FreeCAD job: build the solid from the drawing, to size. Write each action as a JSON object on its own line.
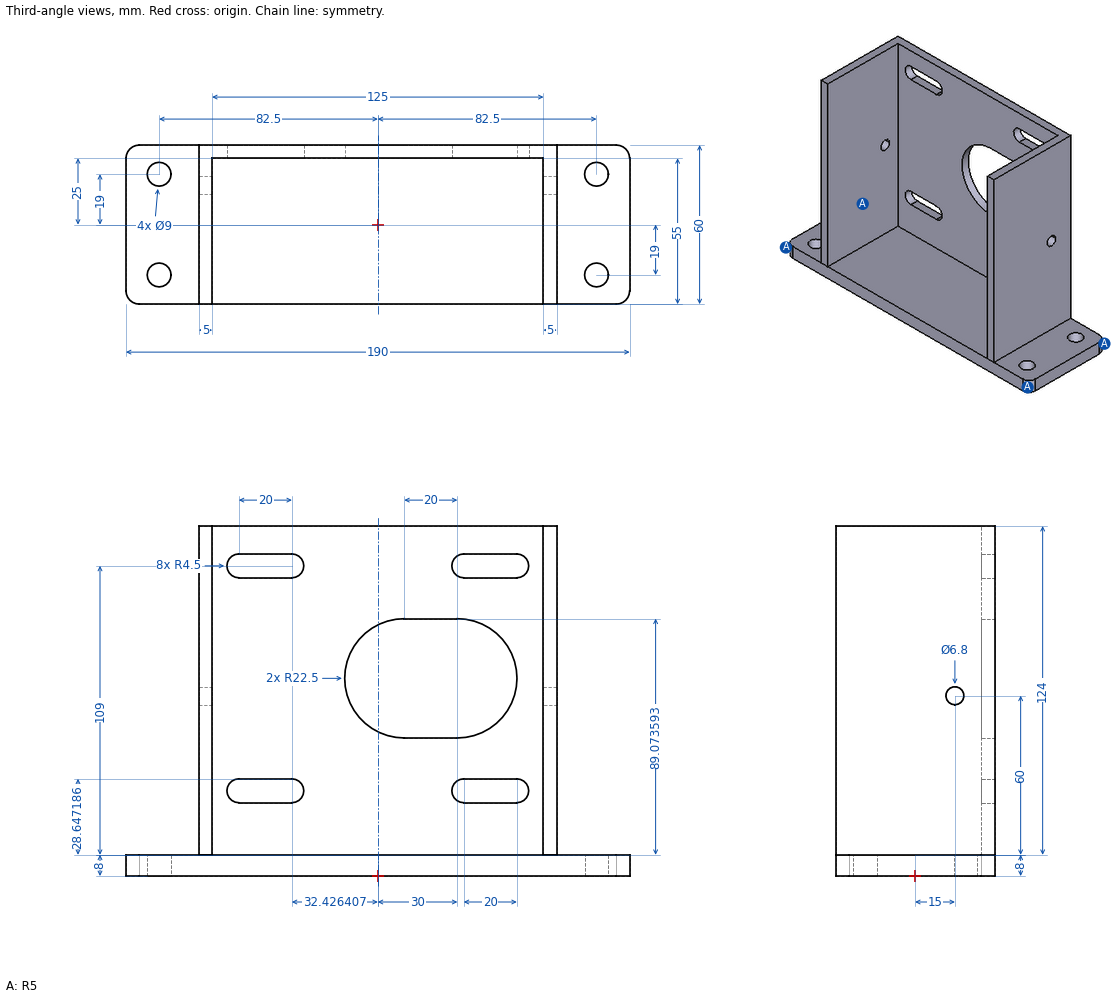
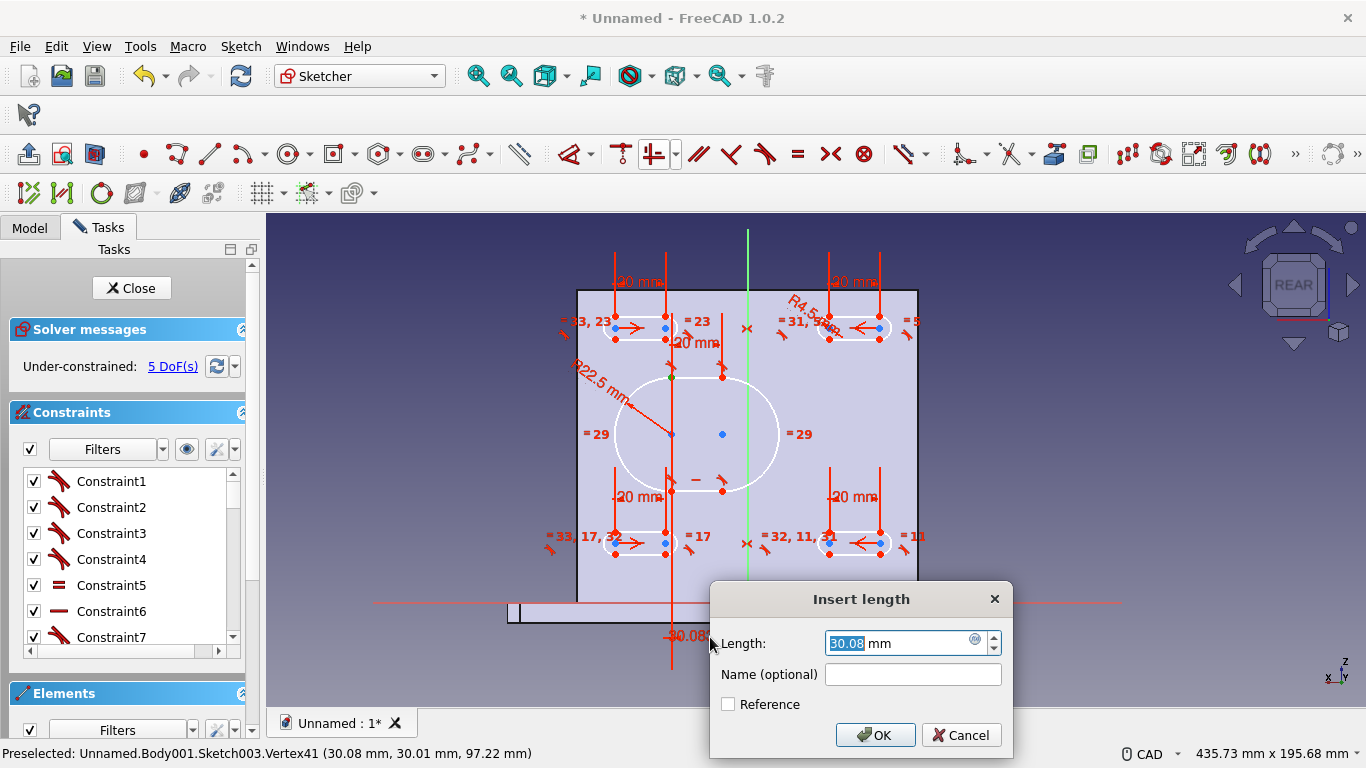
{"action": "type", "text": "30"}
{"action": "key", "text": "Return"}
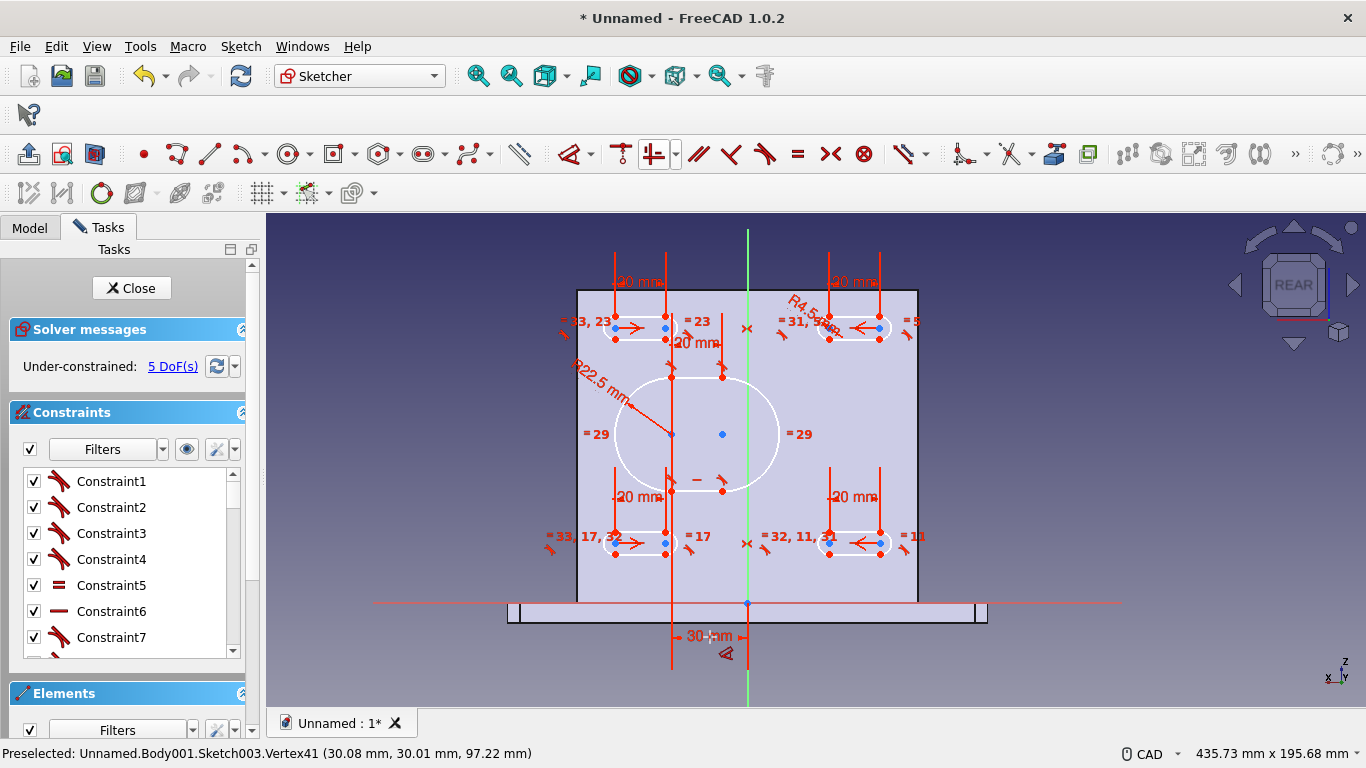
{"action": "left_click", "coordinate": [829, 328]}
{"action": "left_click", "coordinate": [863, 466]}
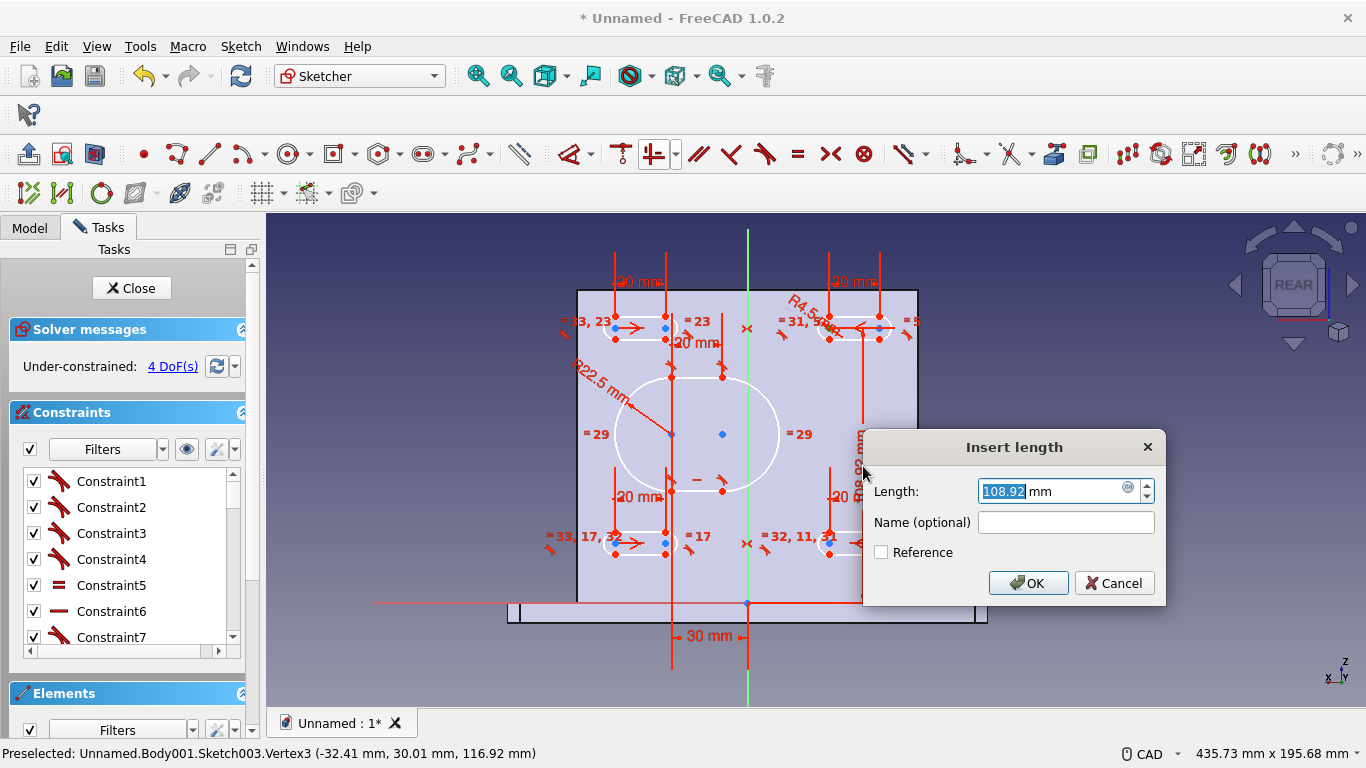
{"action": "type", "text": "109"}
{"action": "key", "text": "Return"}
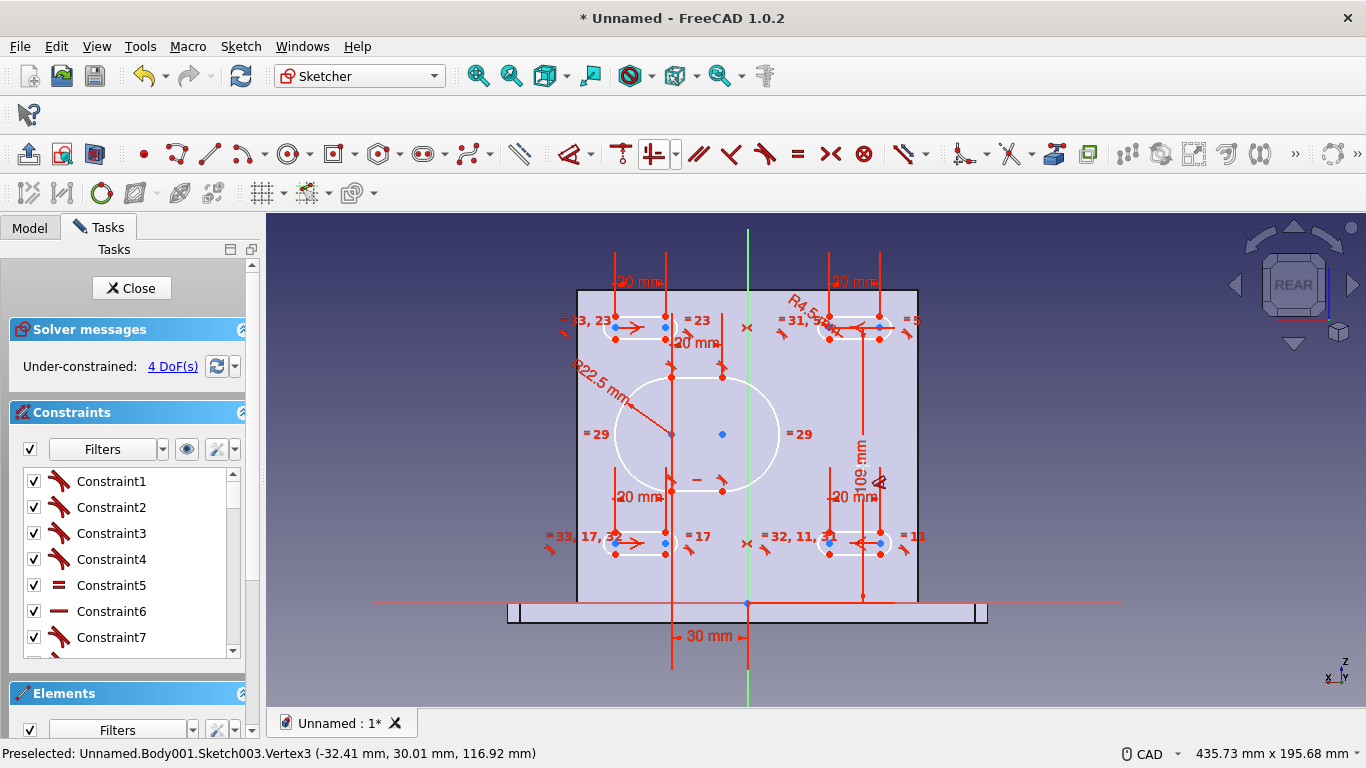
{"action": "left_click", "coordinate": [829, 317]}
{"action": "left_click", "coordinate": [788, 637]}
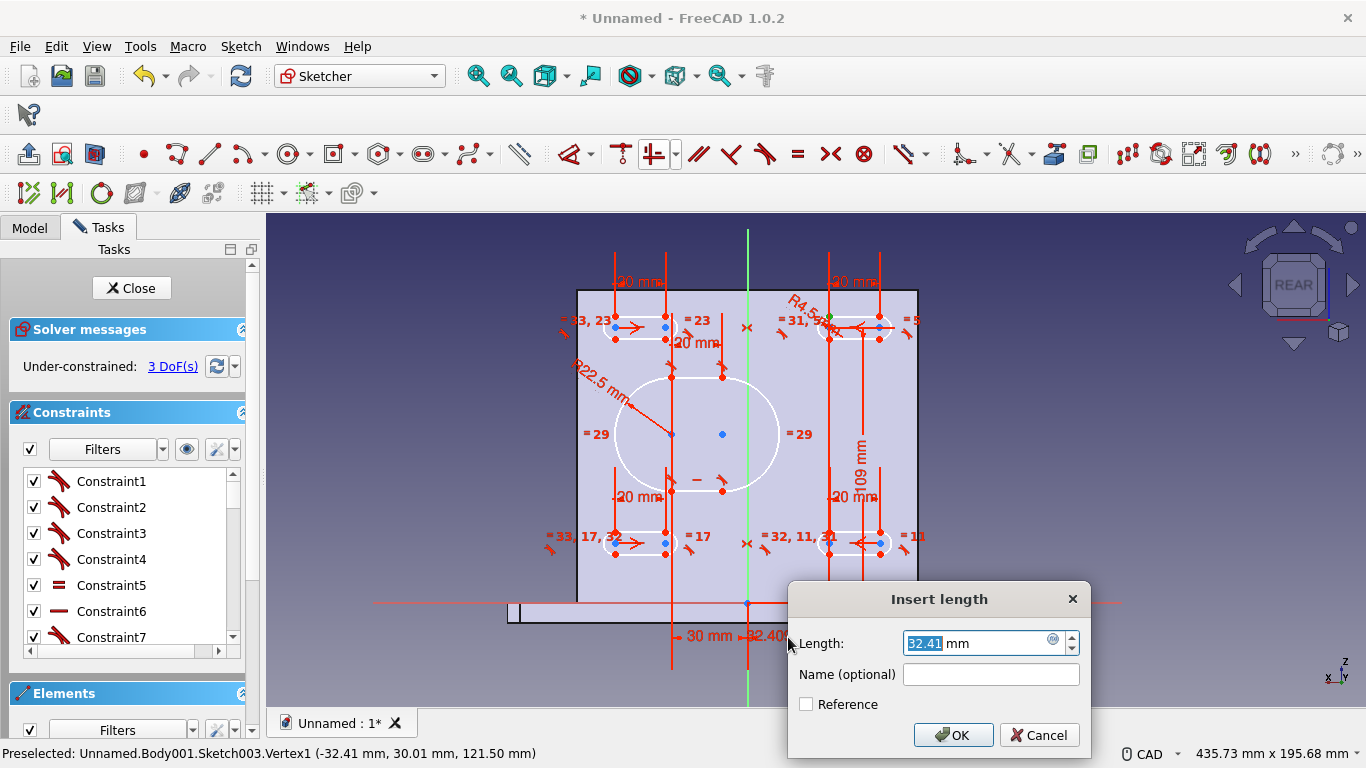
{"action": "type", "text": "32.426407"}
{"action": "key", "text": "Return"}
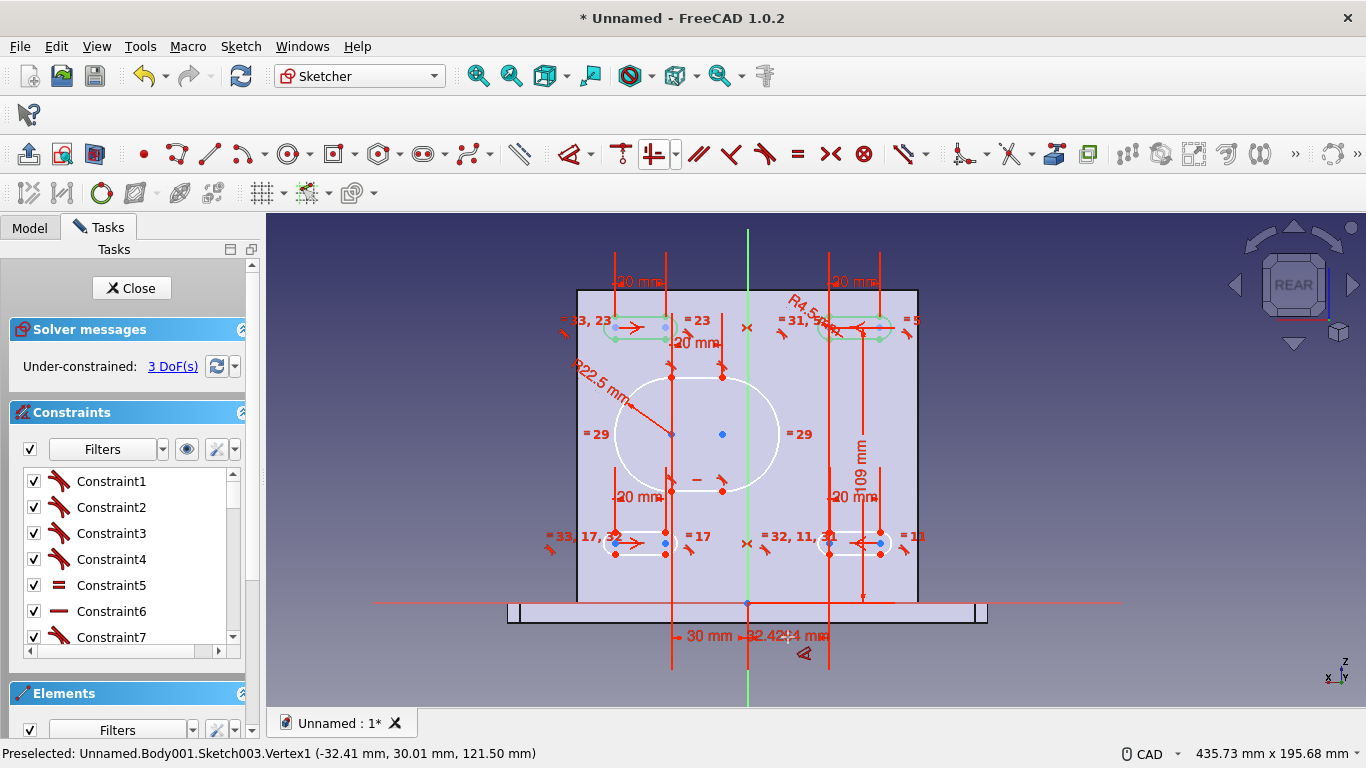
{"action": "left_click", "coordinate": [830, 532]}
{"action": "left_click", "coordinate": [770, 498]}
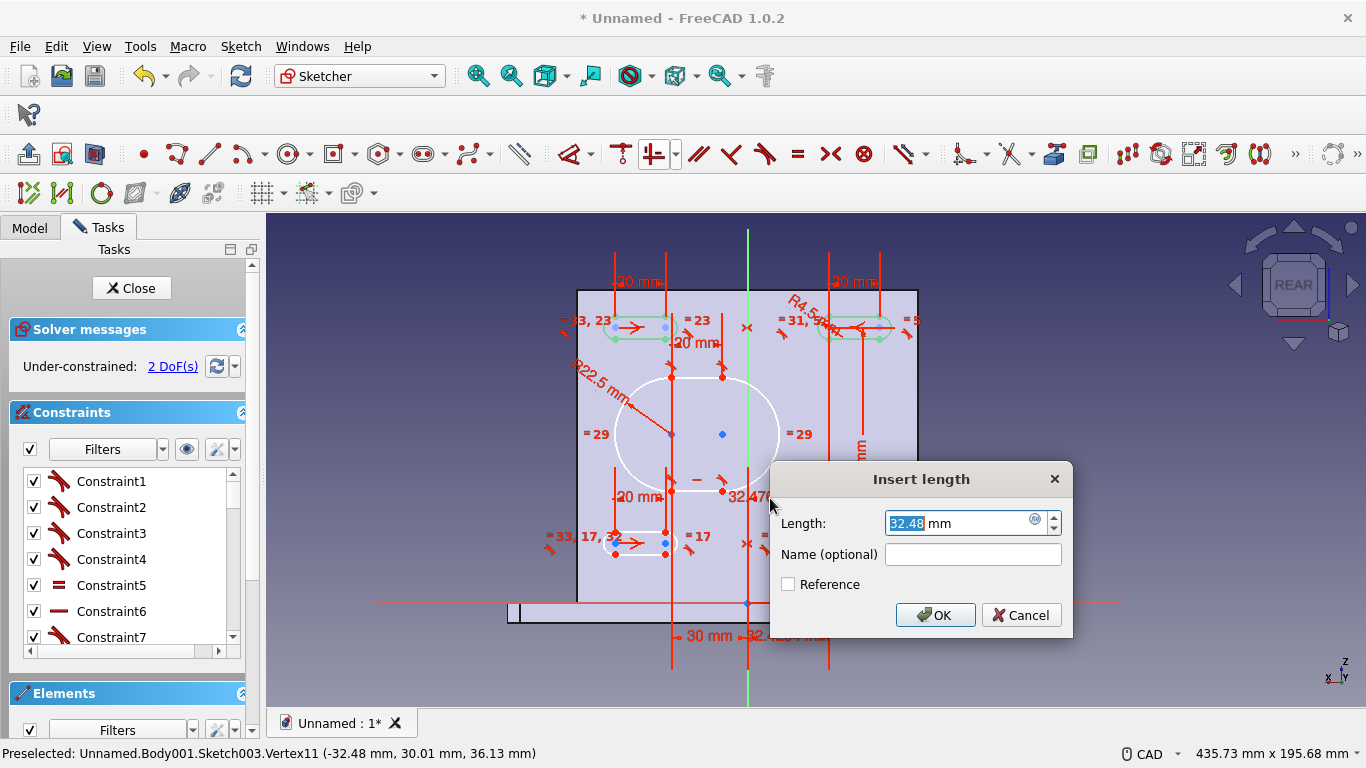
{"action": "type", "text": "32.426407"}
{"action": "key", "text": "Return"}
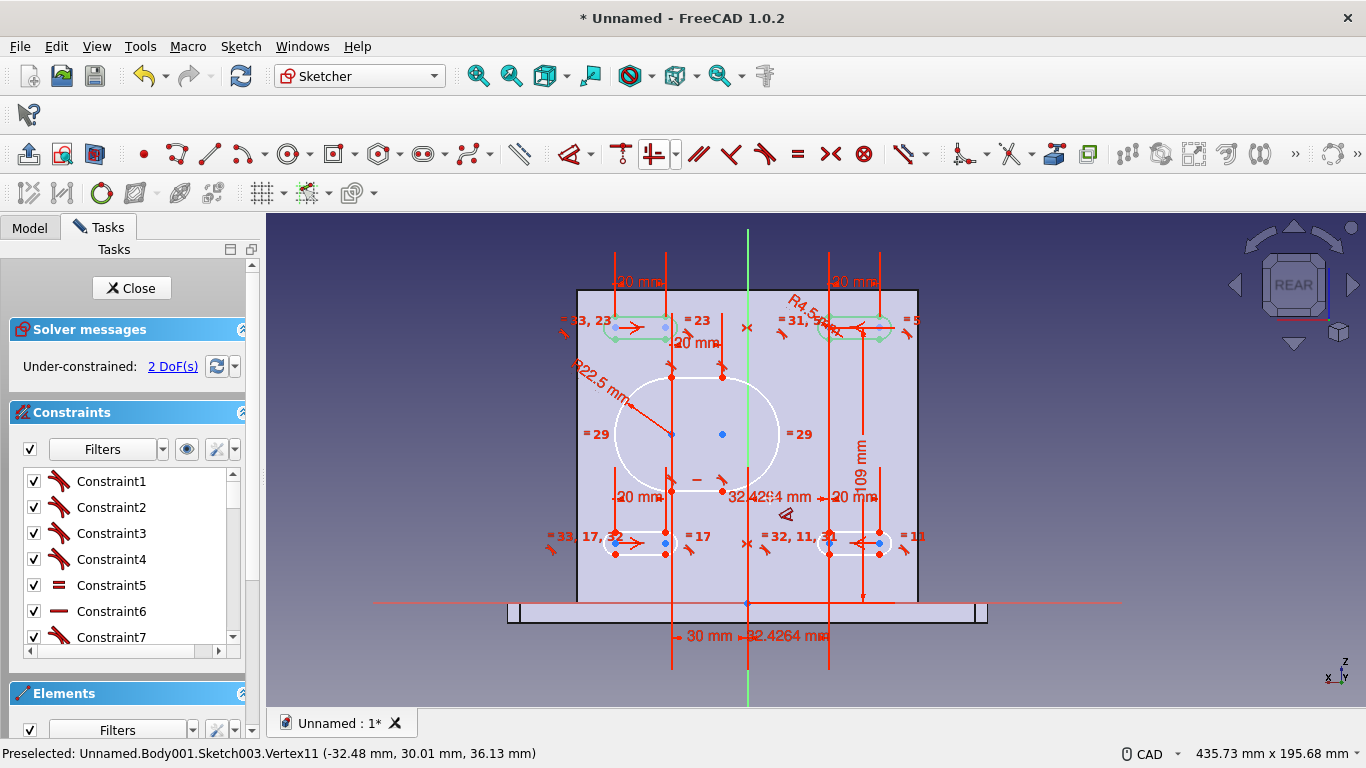
{"action": "left_click", "coordinate": [829, 532]}
{"action": "left_click", "coordinate": [863, 584]}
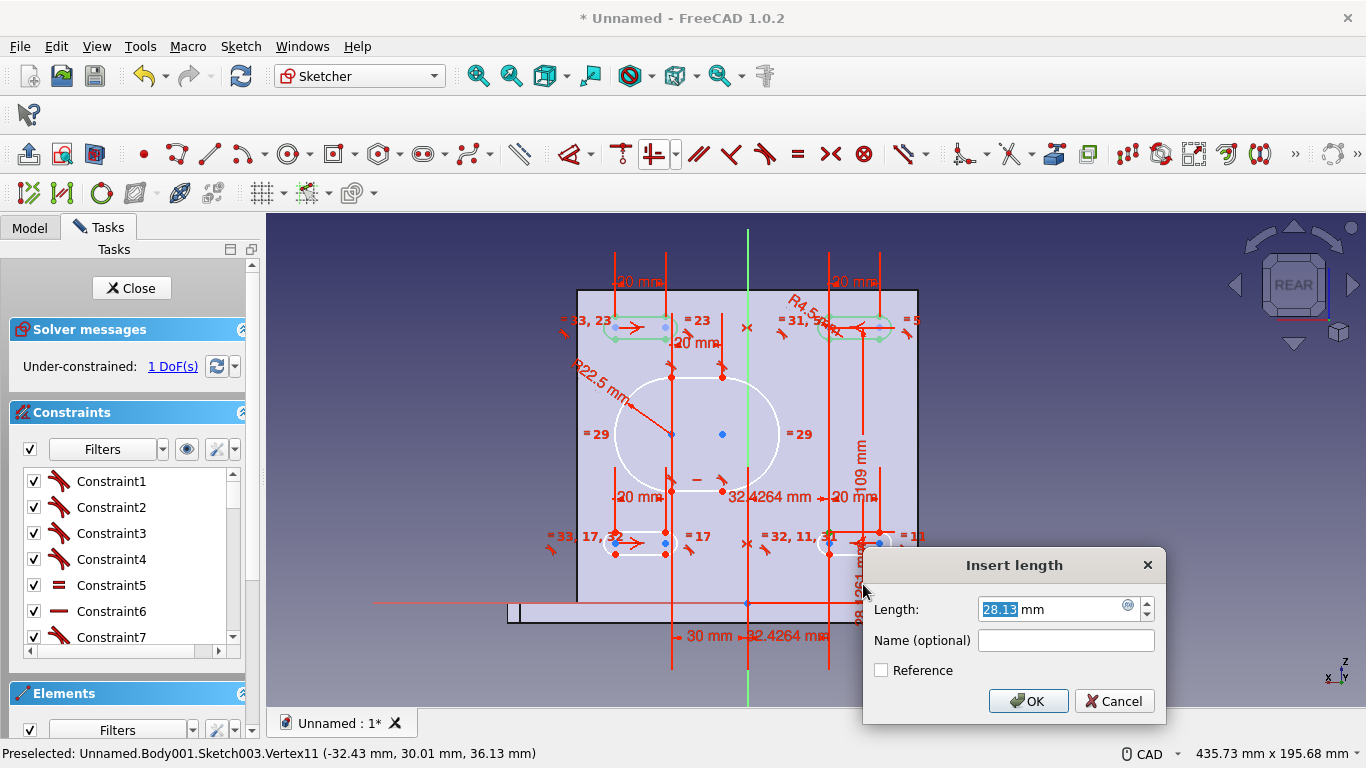
{"action": "type", "text": "28.647186"}
{"action": "key", "text": "Return"}